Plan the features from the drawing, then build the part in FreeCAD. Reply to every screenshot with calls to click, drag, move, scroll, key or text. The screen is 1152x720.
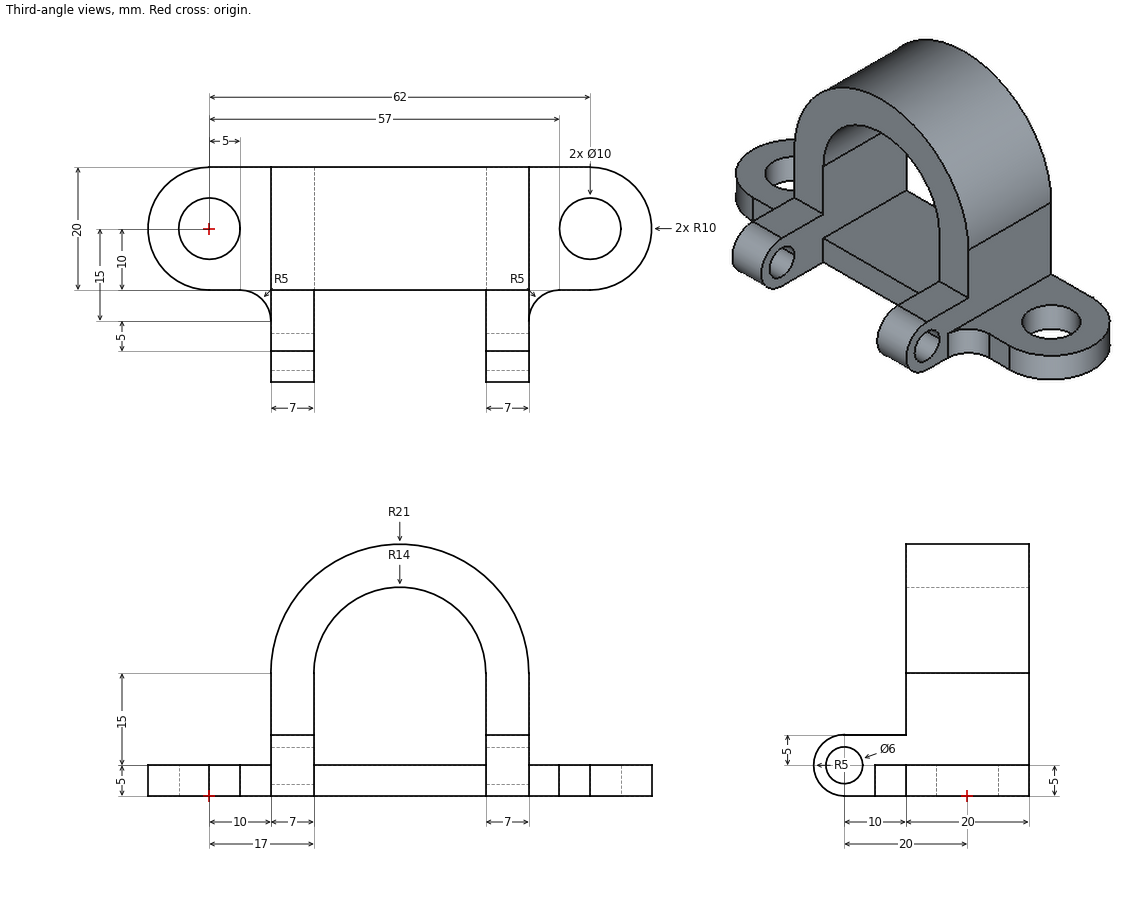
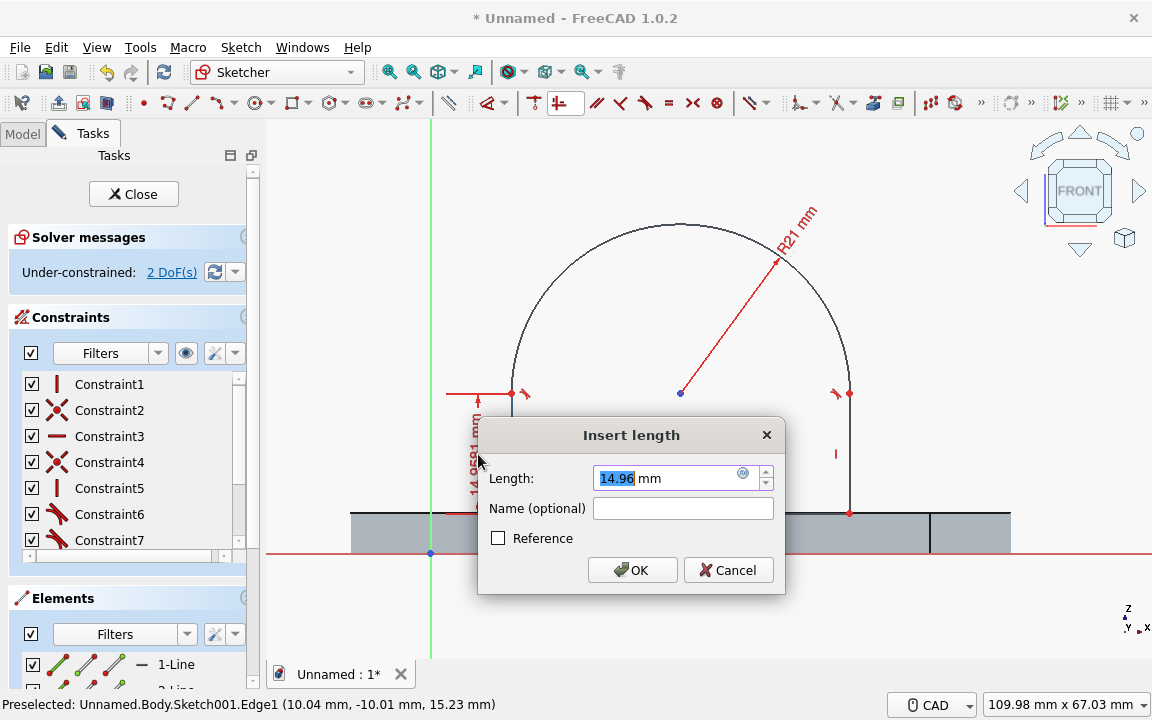
text(15)
key(Return)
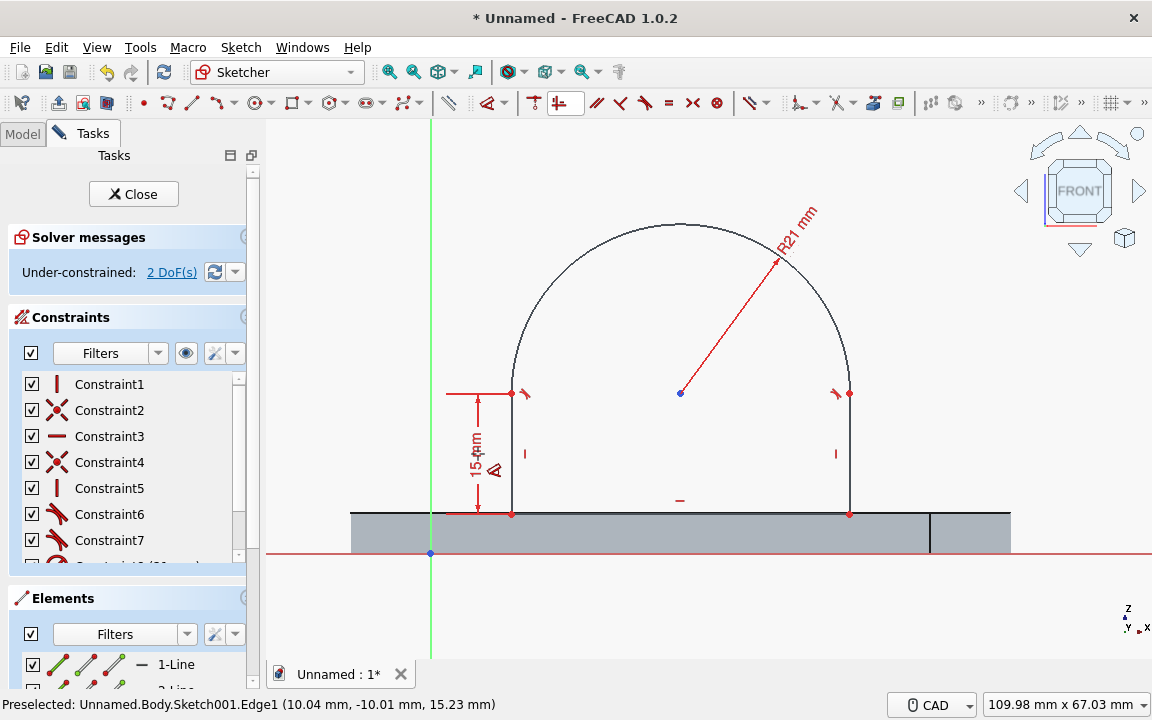
click(512, 514)
click(397, 534)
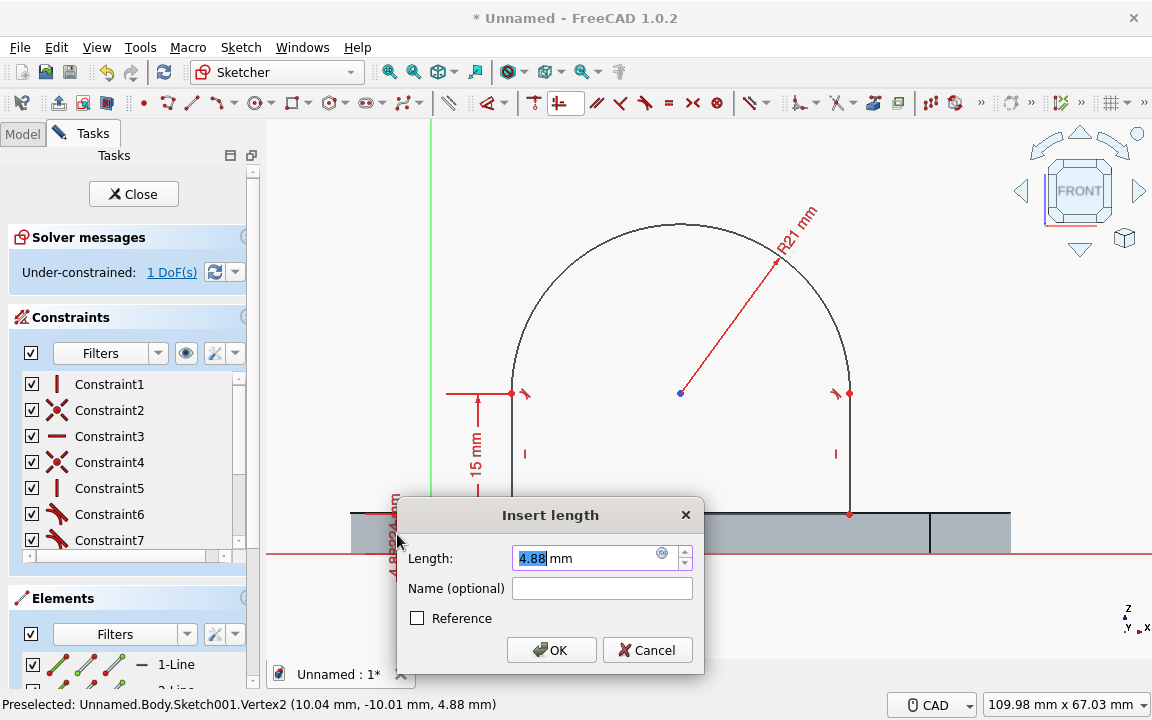
text(5)
key(Return)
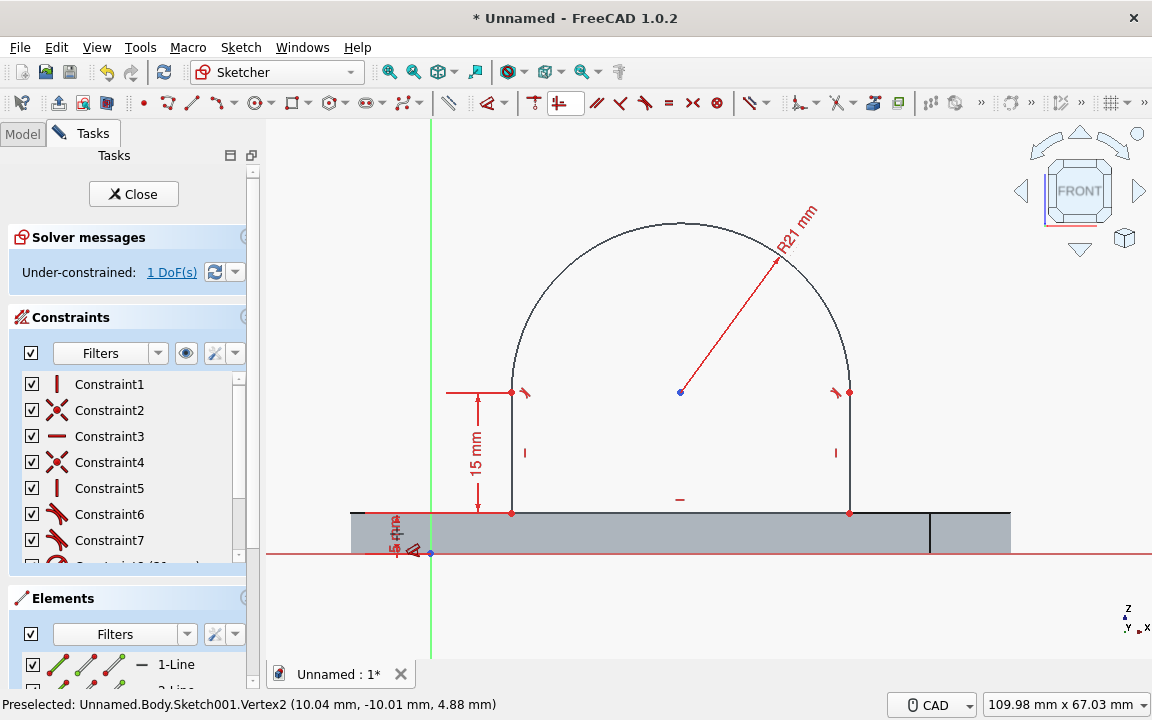
click(512, 393)
click(471, 588)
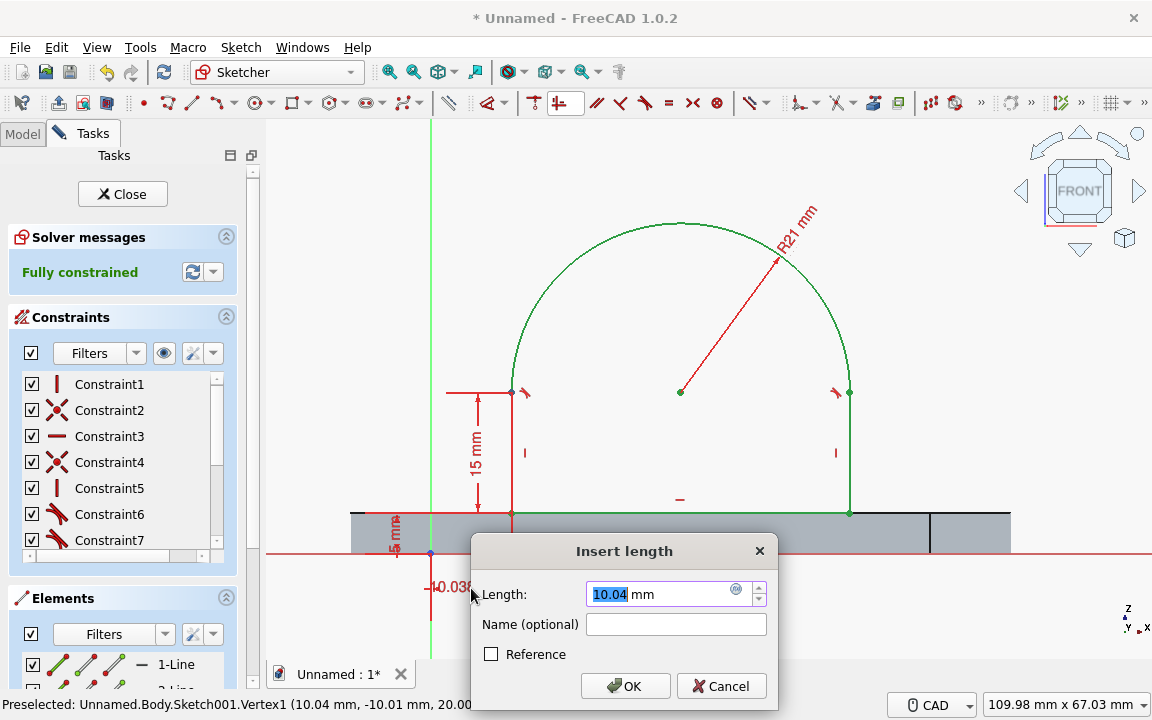
text(10)
key(Return)
key(Escape)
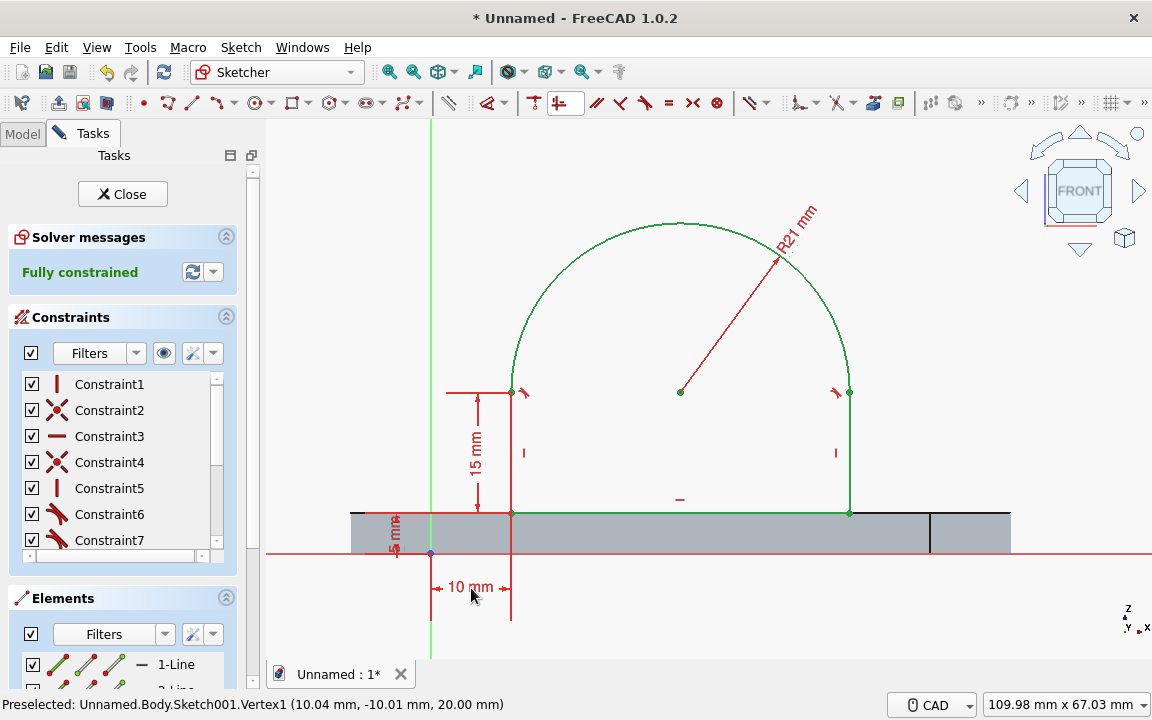
click(123, 194)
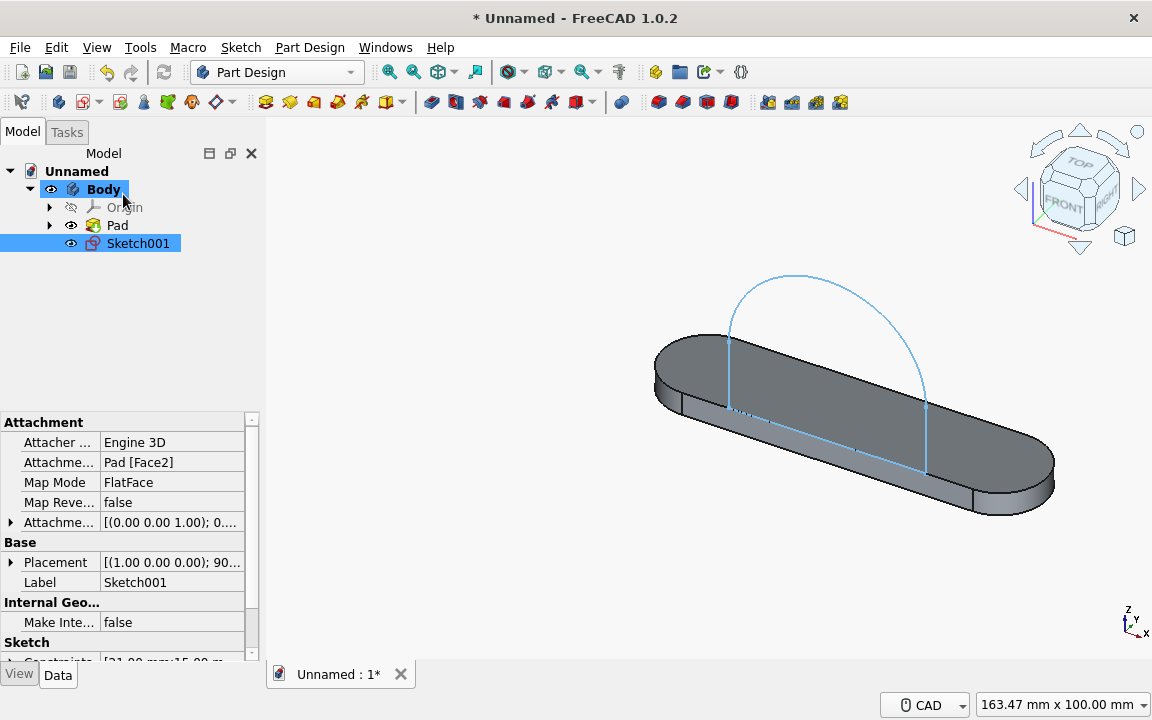
click(266, 102)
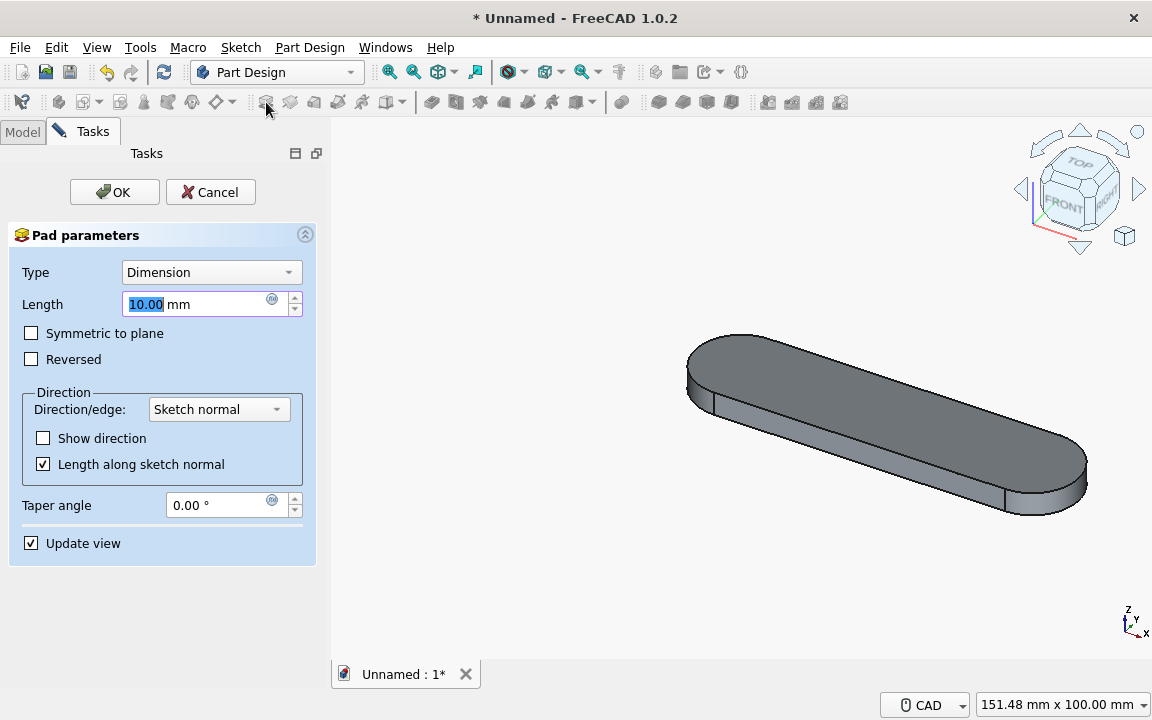
text(20)
key(Tab)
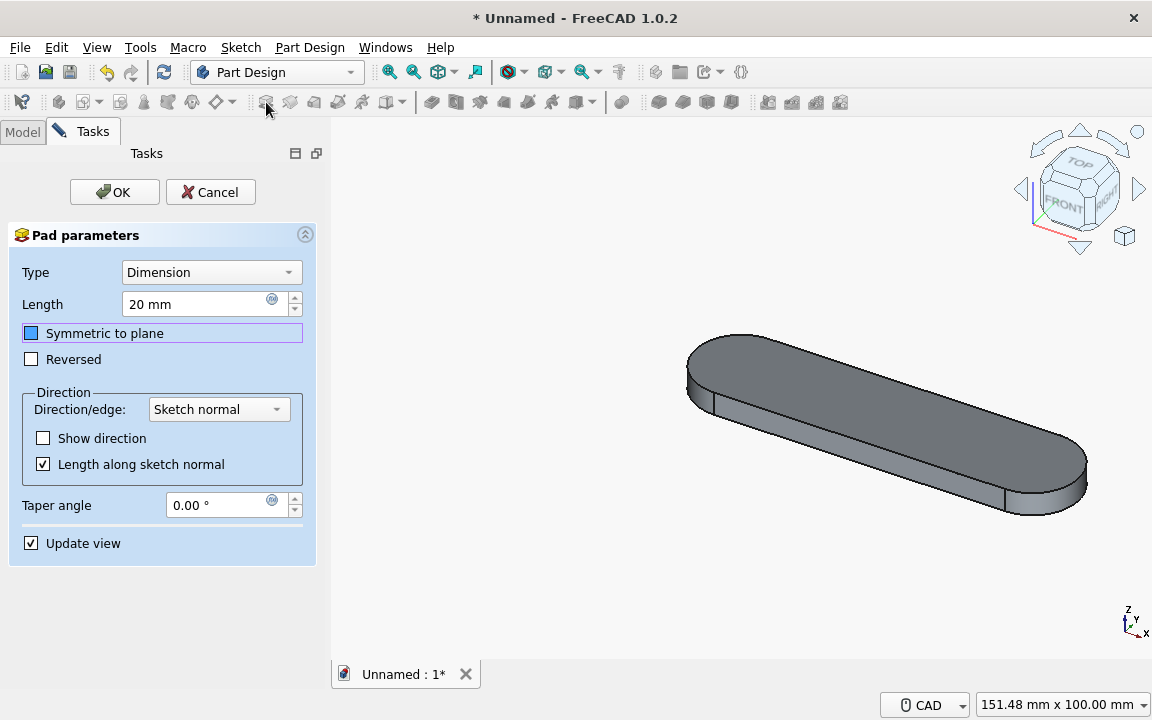
click(30, 359)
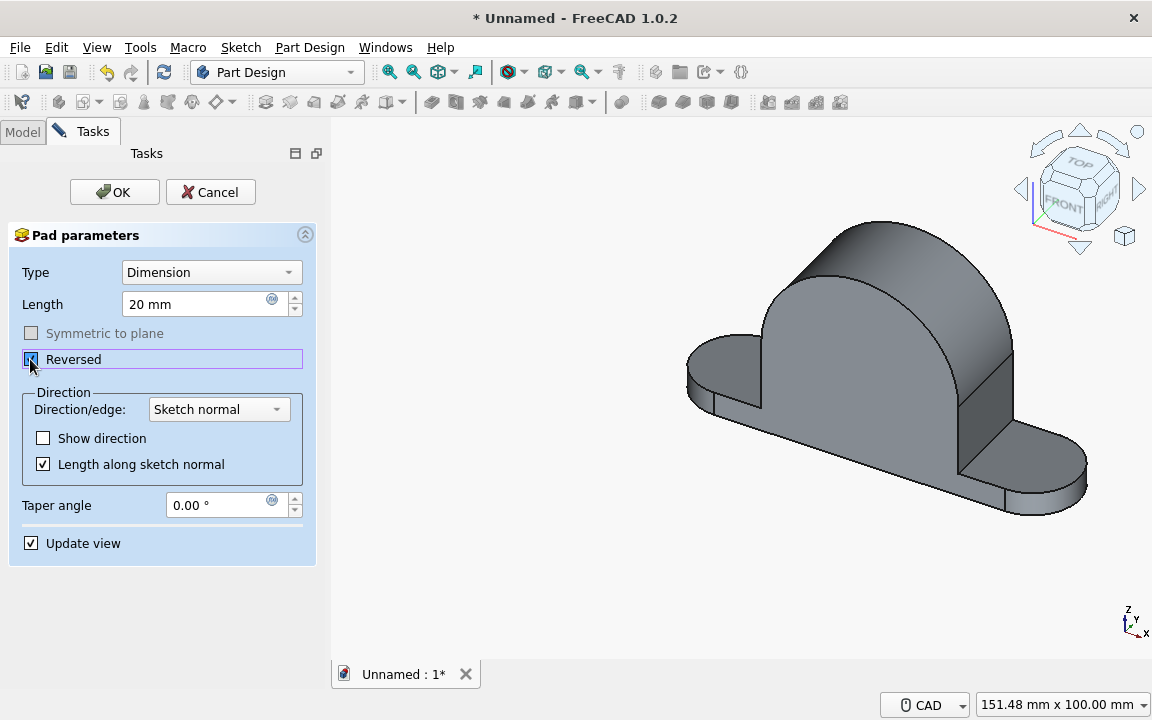
click(115, 192)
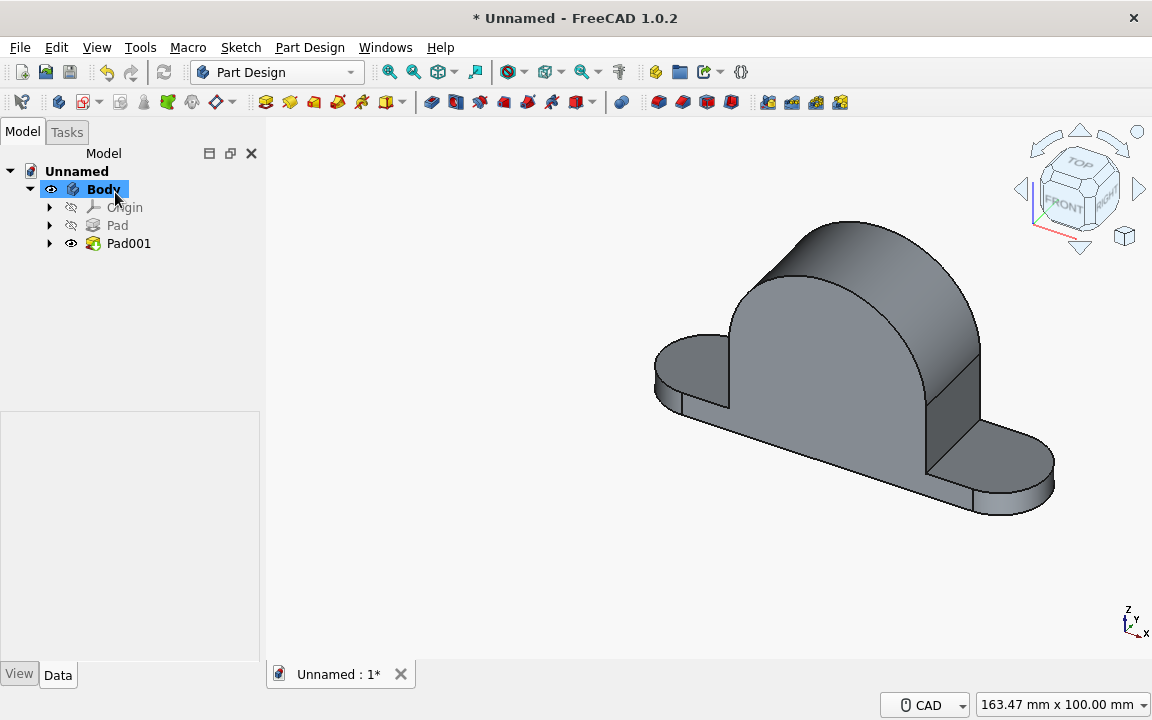
click(827, 371)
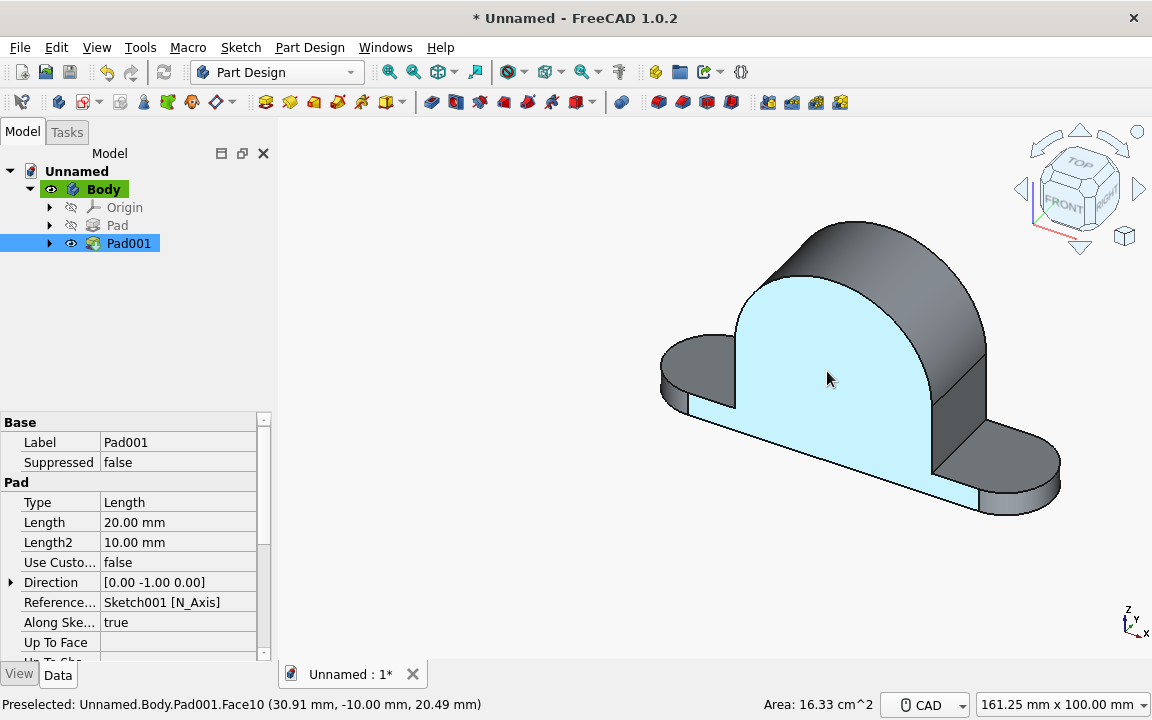
click(84, 102)